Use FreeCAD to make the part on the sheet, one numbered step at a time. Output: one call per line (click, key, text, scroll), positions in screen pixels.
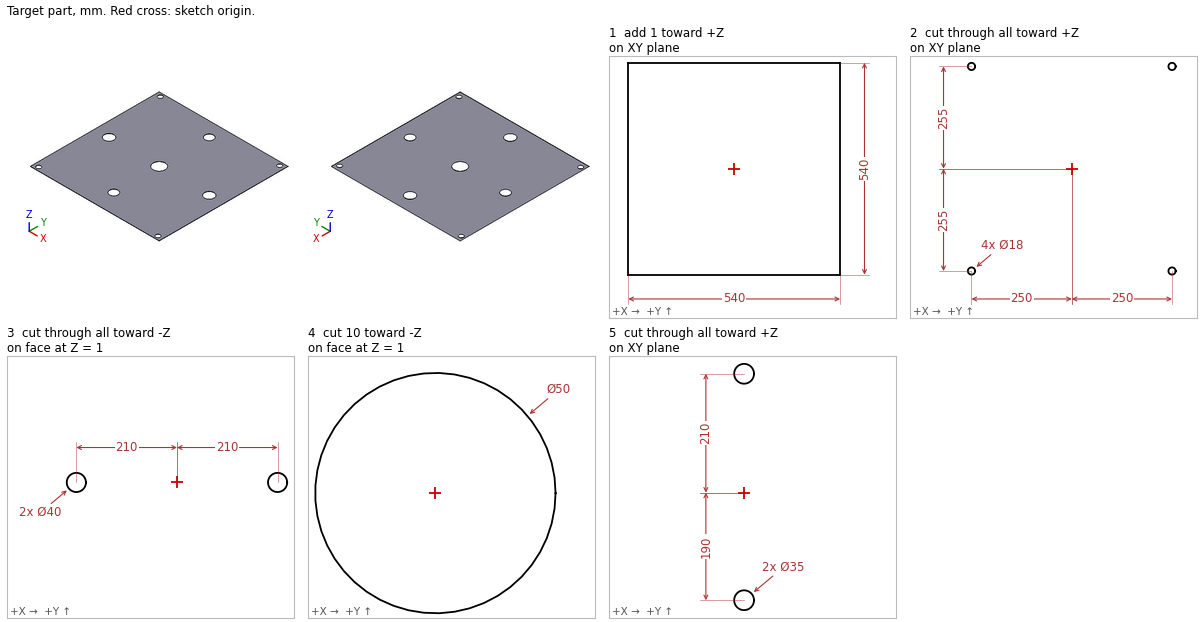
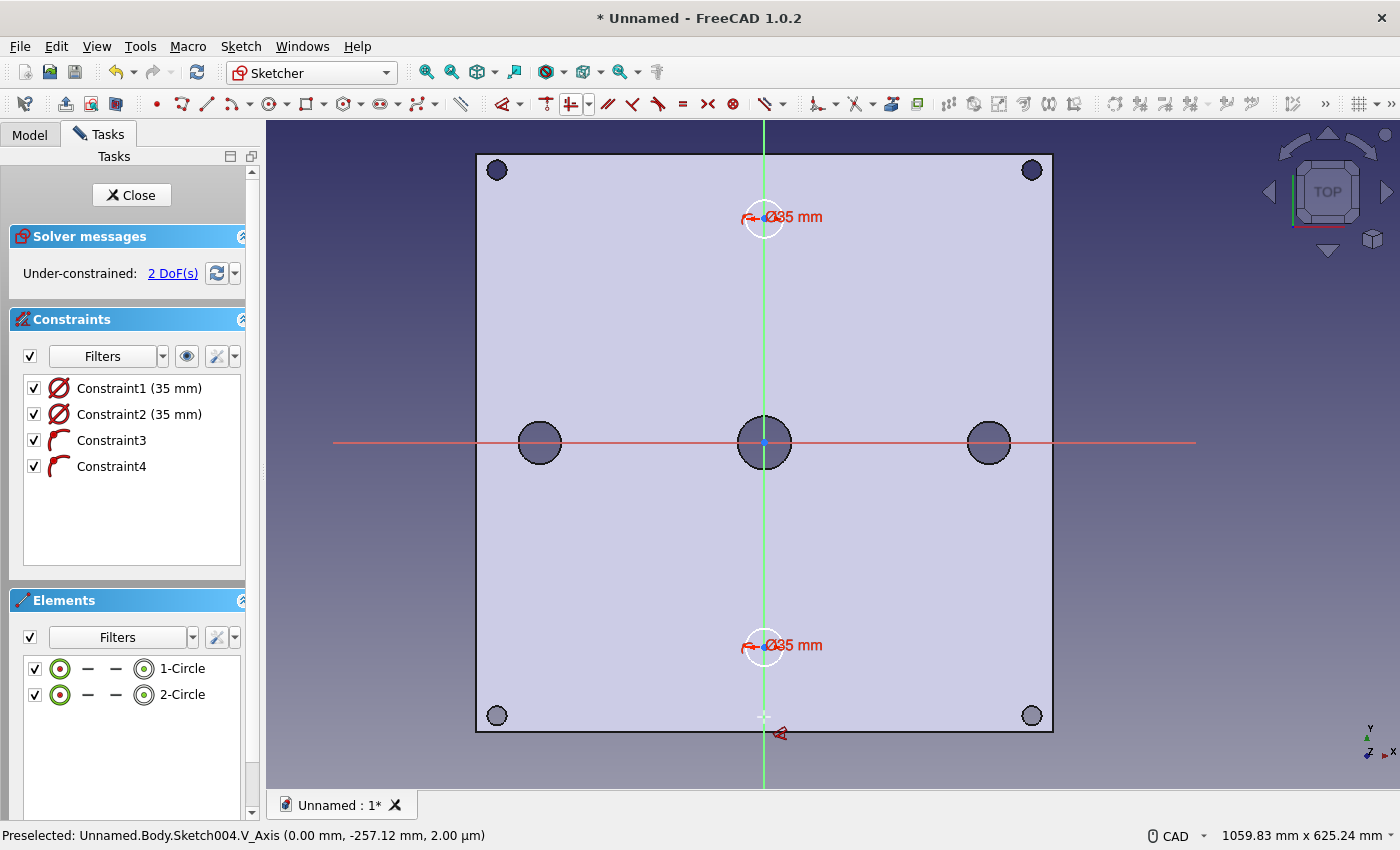
click(764, 647)
click(798, 545)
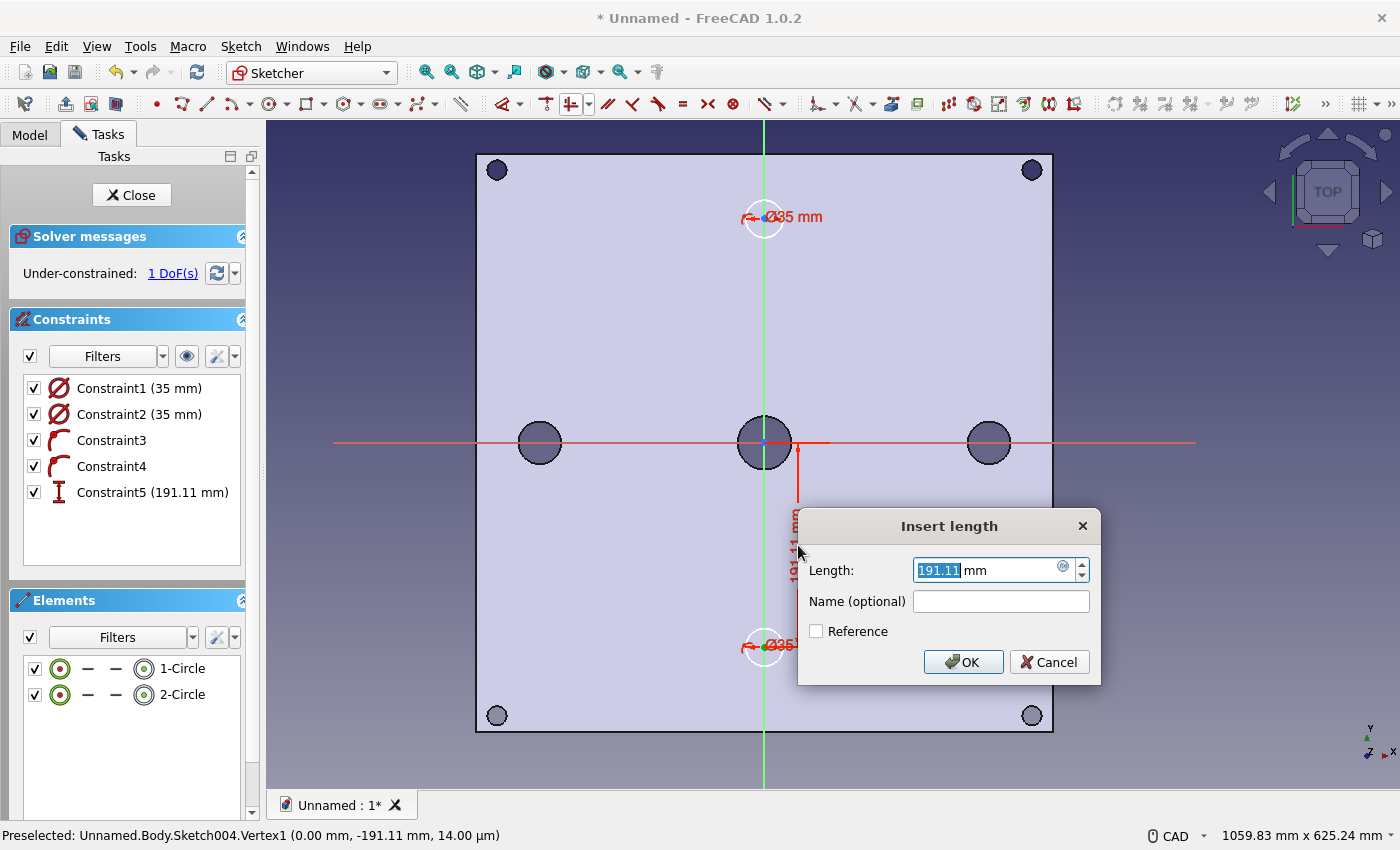
text(190)
key(Return)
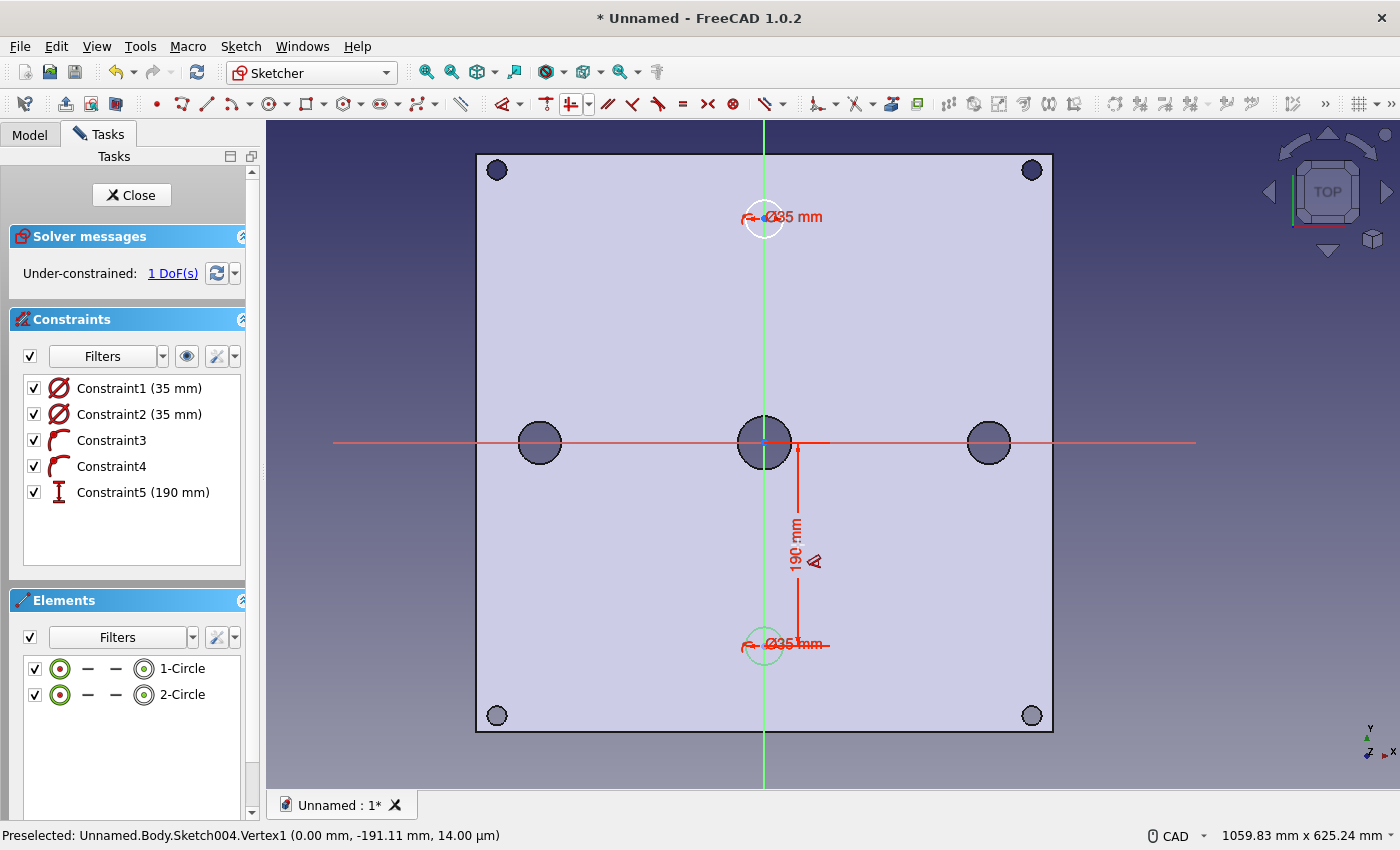
click(764, 219)
click(798, 331)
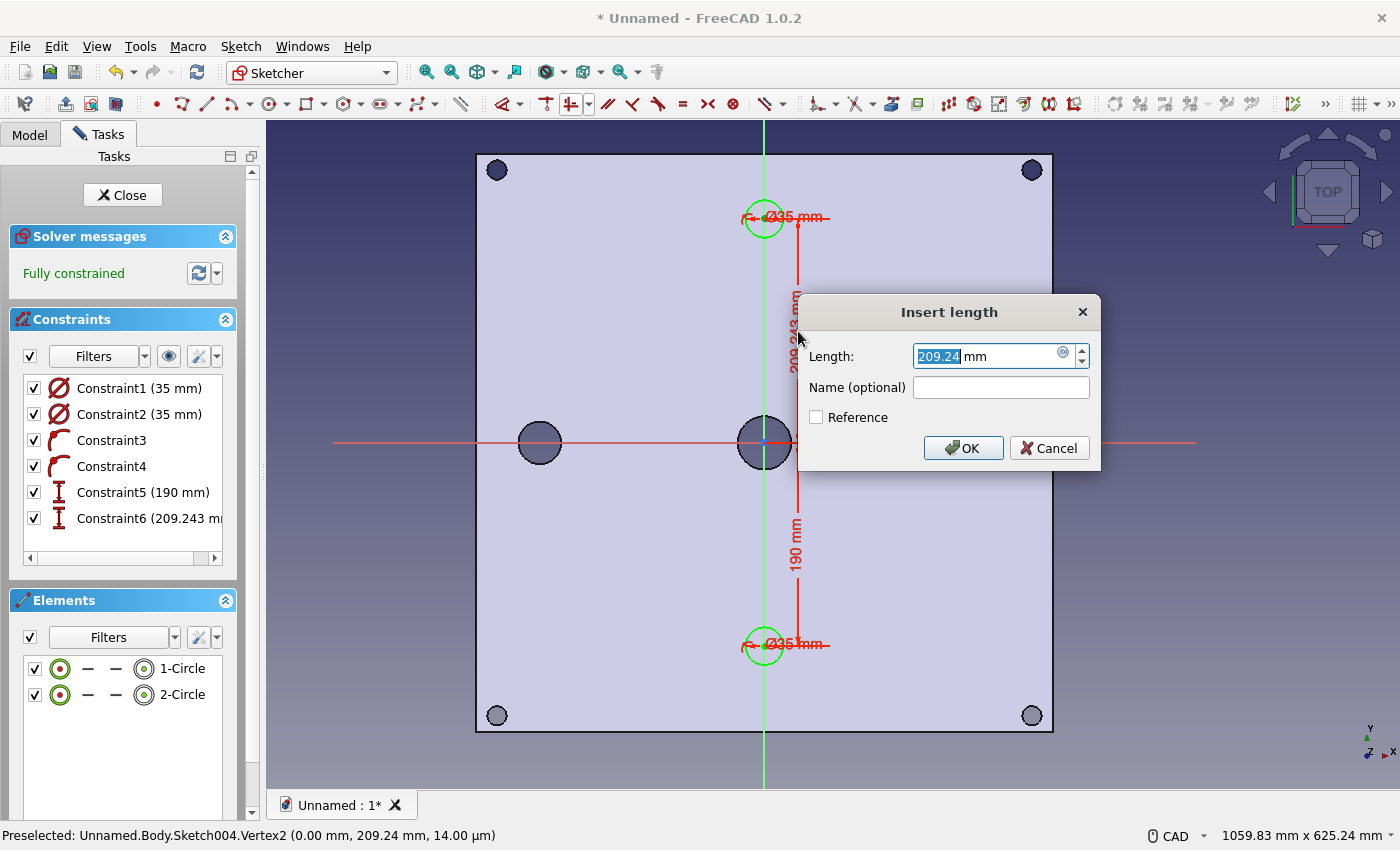
text(210)
key(Return)
key(Escape)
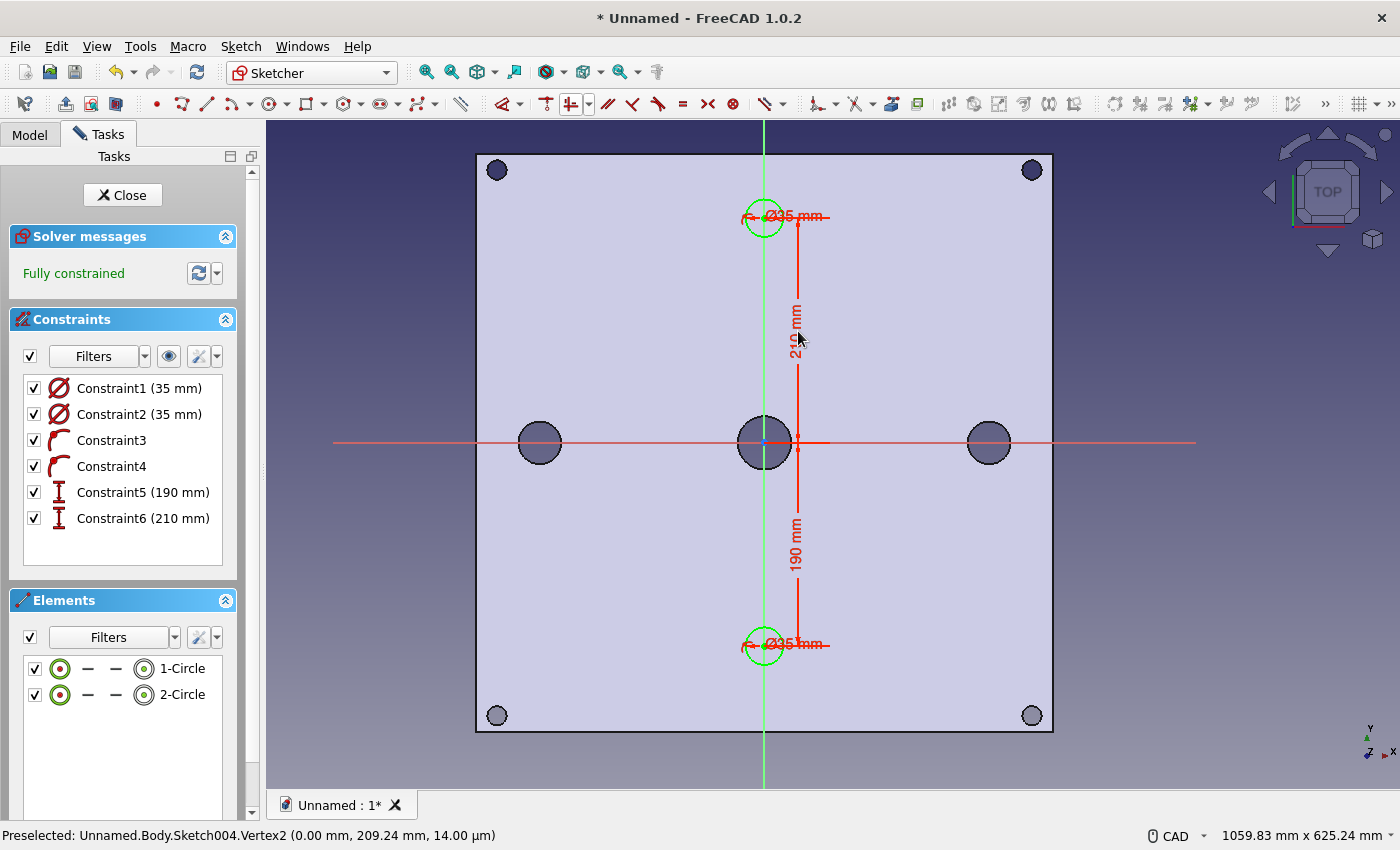
click(123, 195)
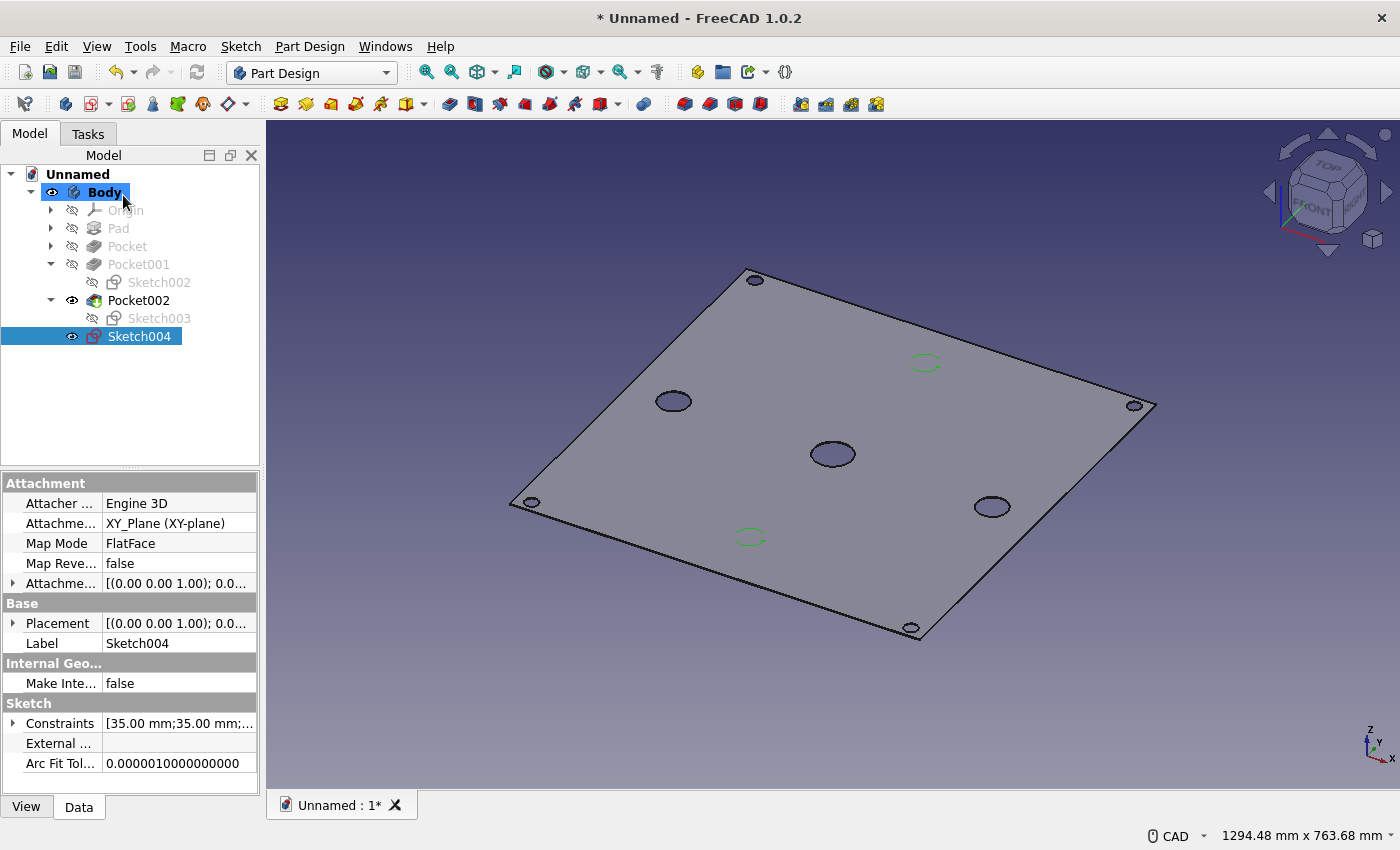
click(450, 104)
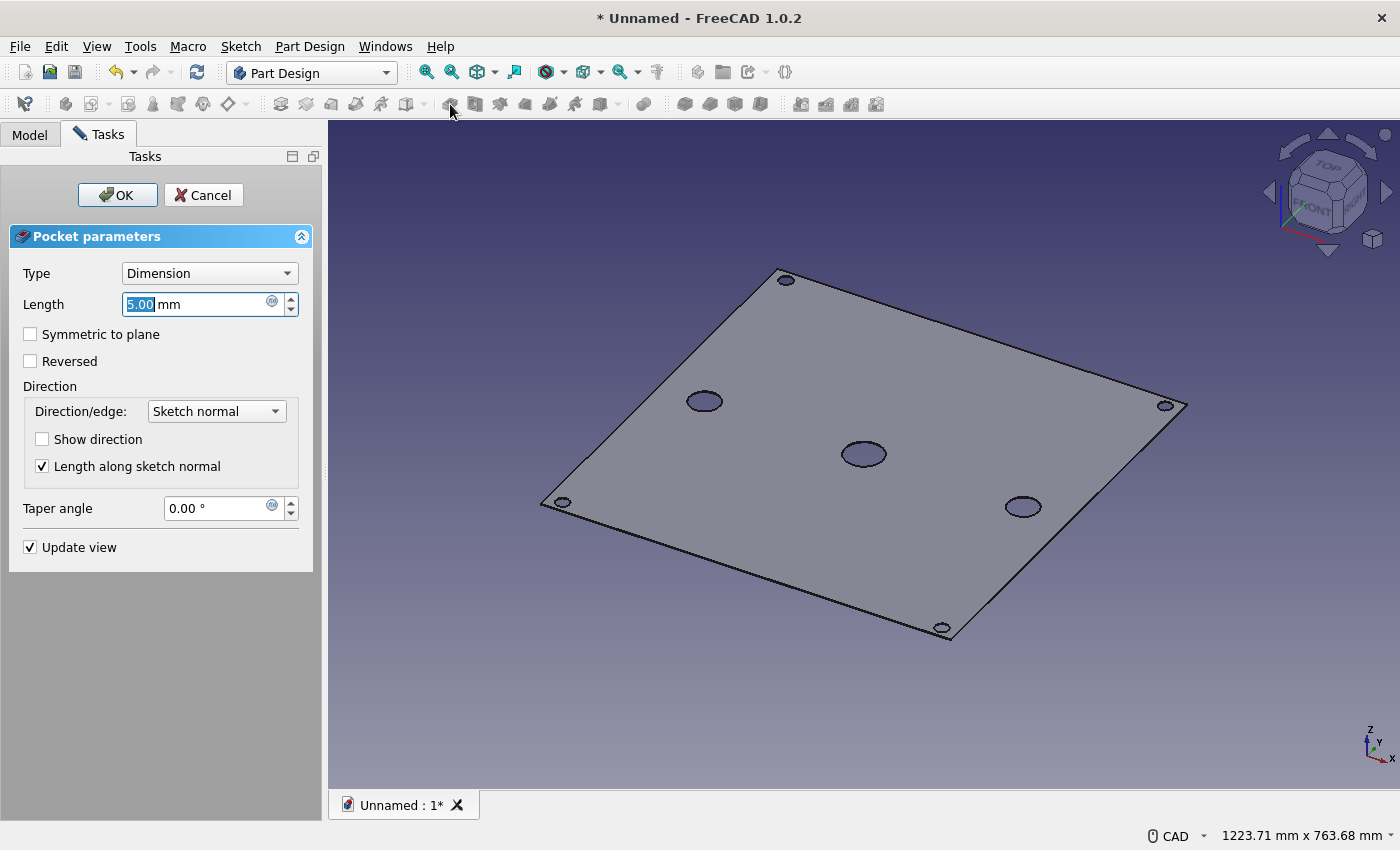
click(210, 274)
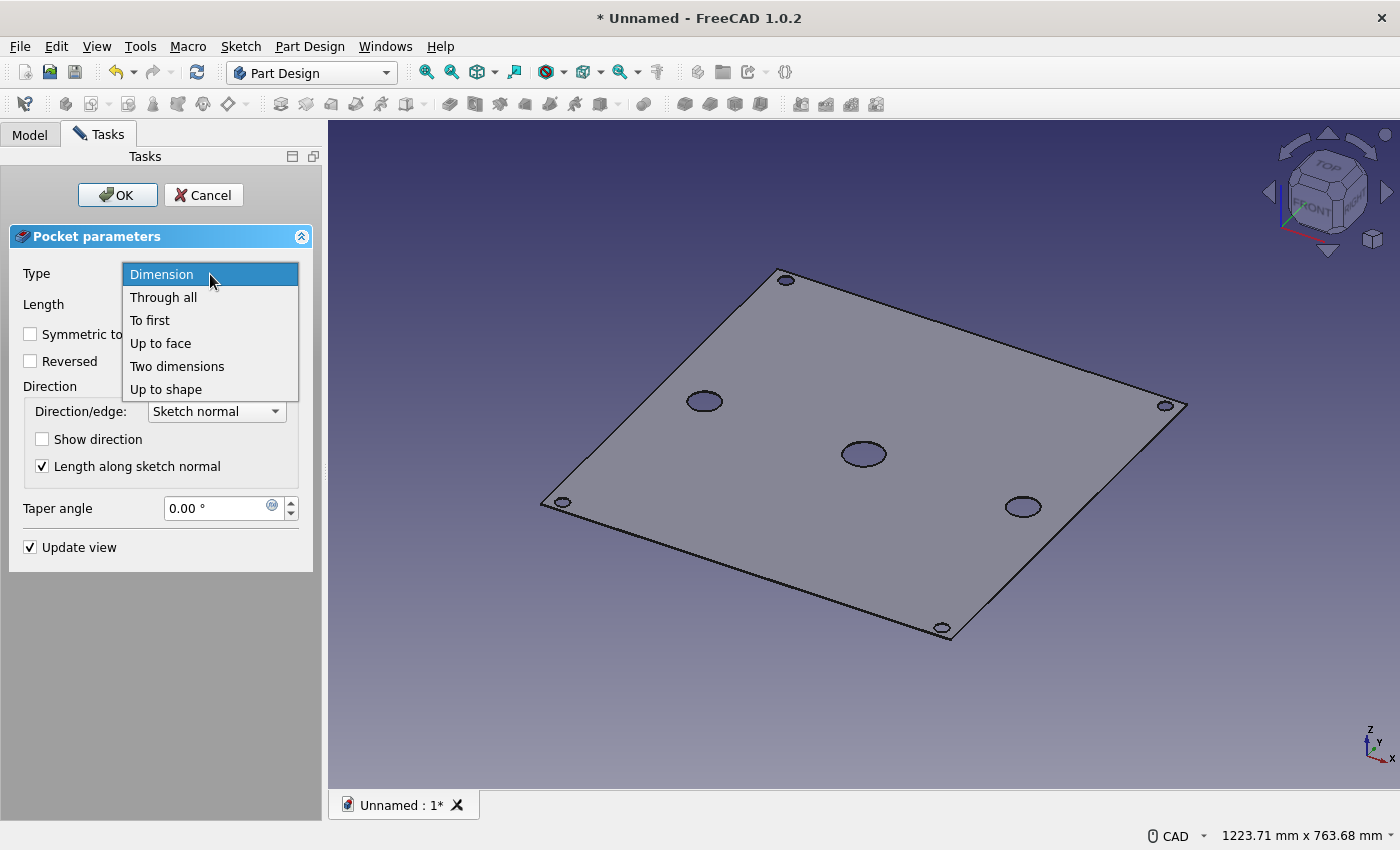
click(208, 298)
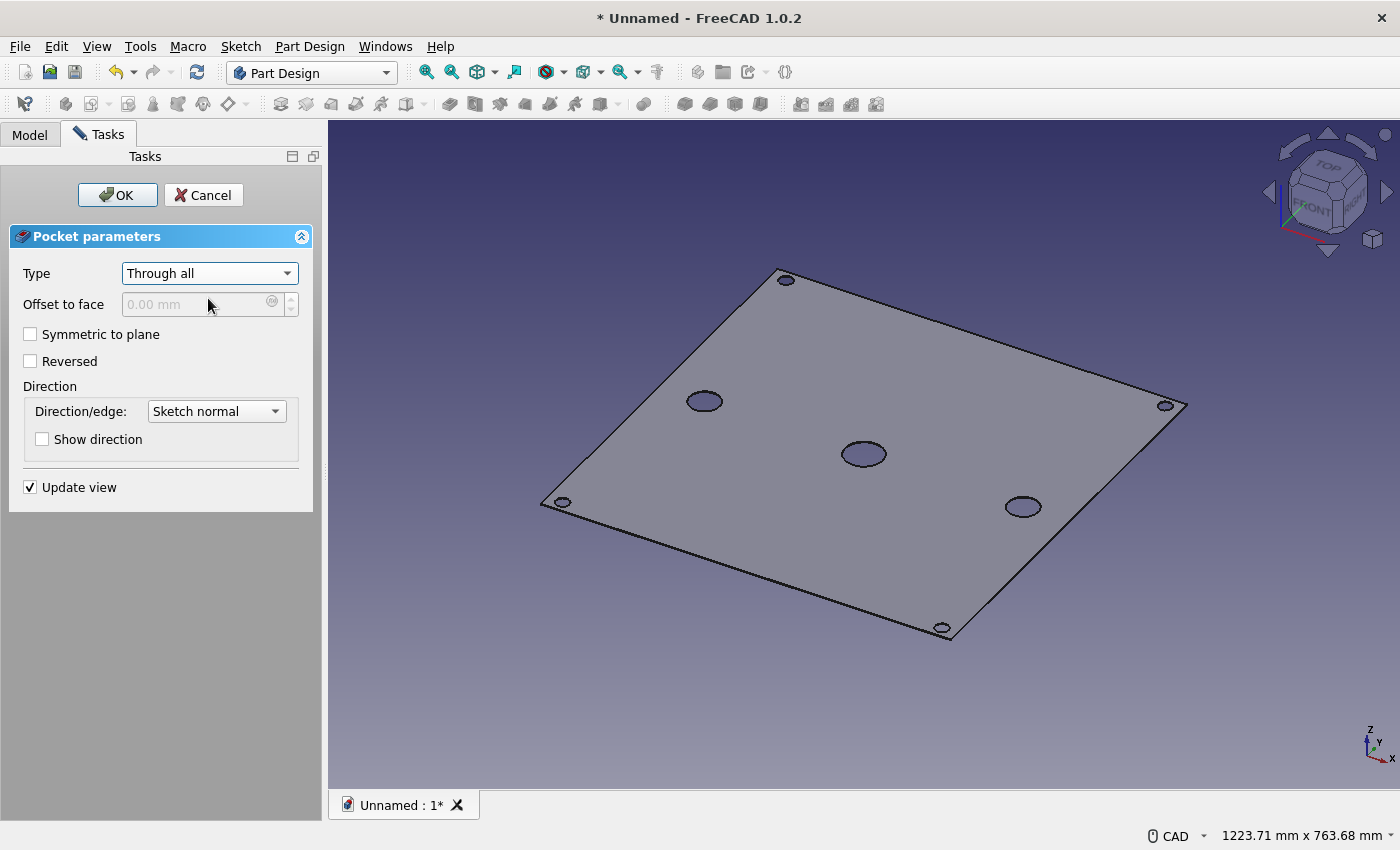
click(31, 361)